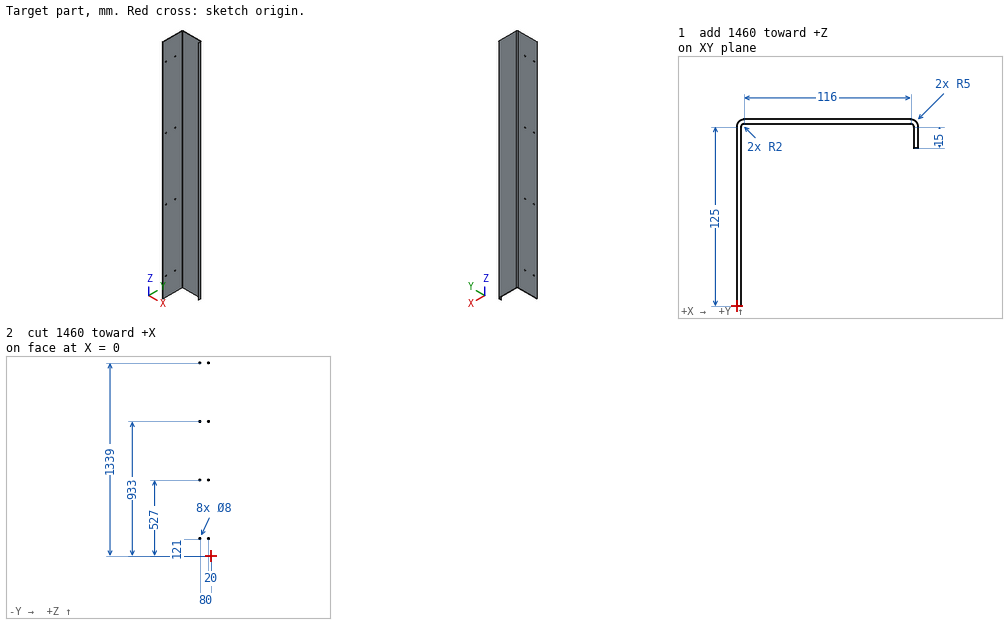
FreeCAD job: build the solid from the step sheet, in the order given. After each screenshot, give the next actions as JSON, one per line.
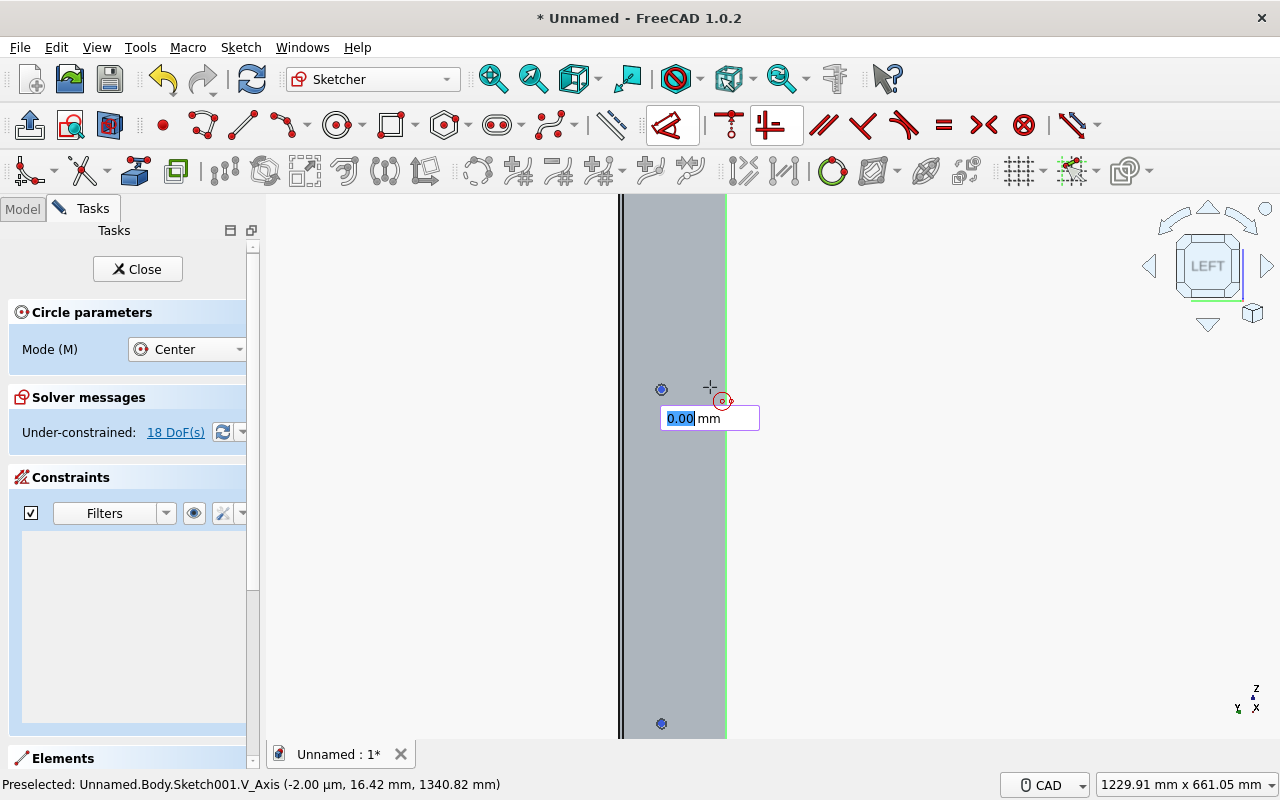
{"action": "scroll", "coordinate": [712, 384], "scroll_direction": "up", "scroll_amount": 8}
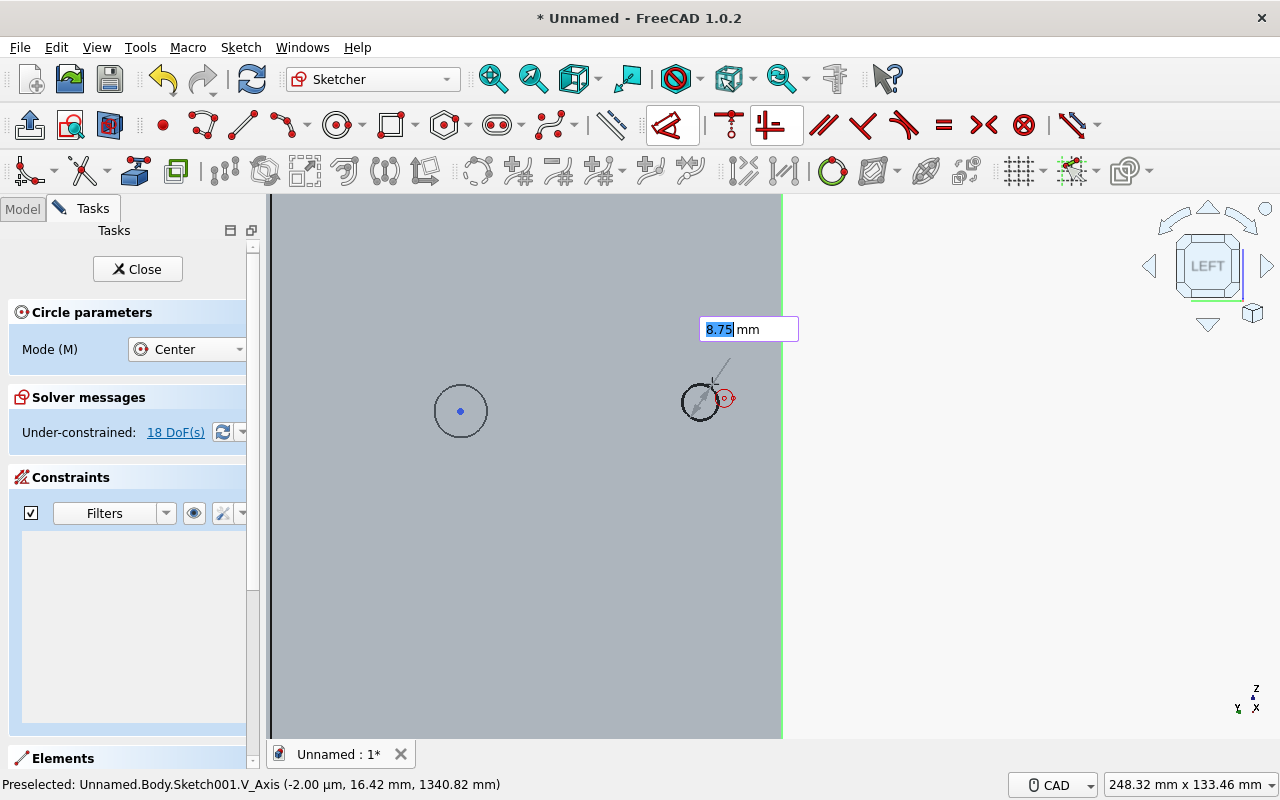
{"action": "left_click", "coordinate": [712, 385]}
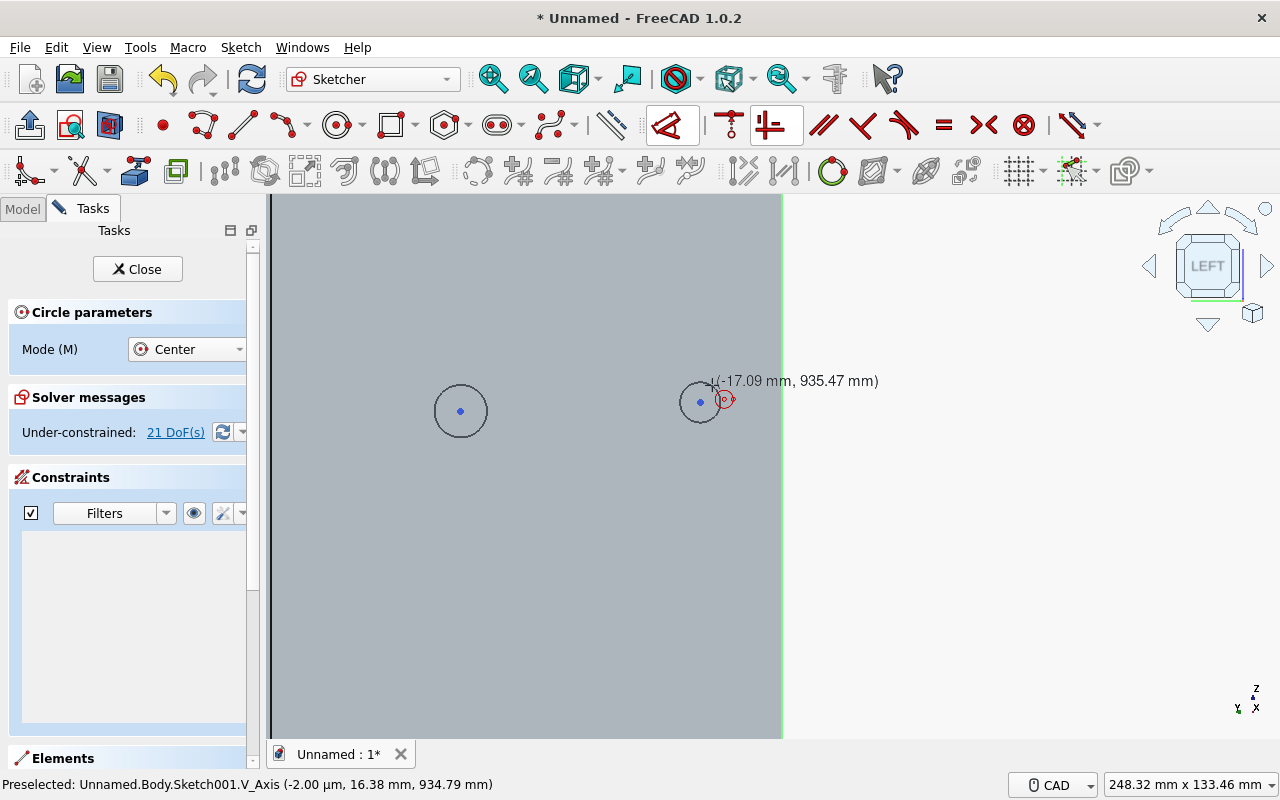
{"action": "scroll", "coordinate": [711, 402], "scroll_direction": "down", "scroll_amount": 14}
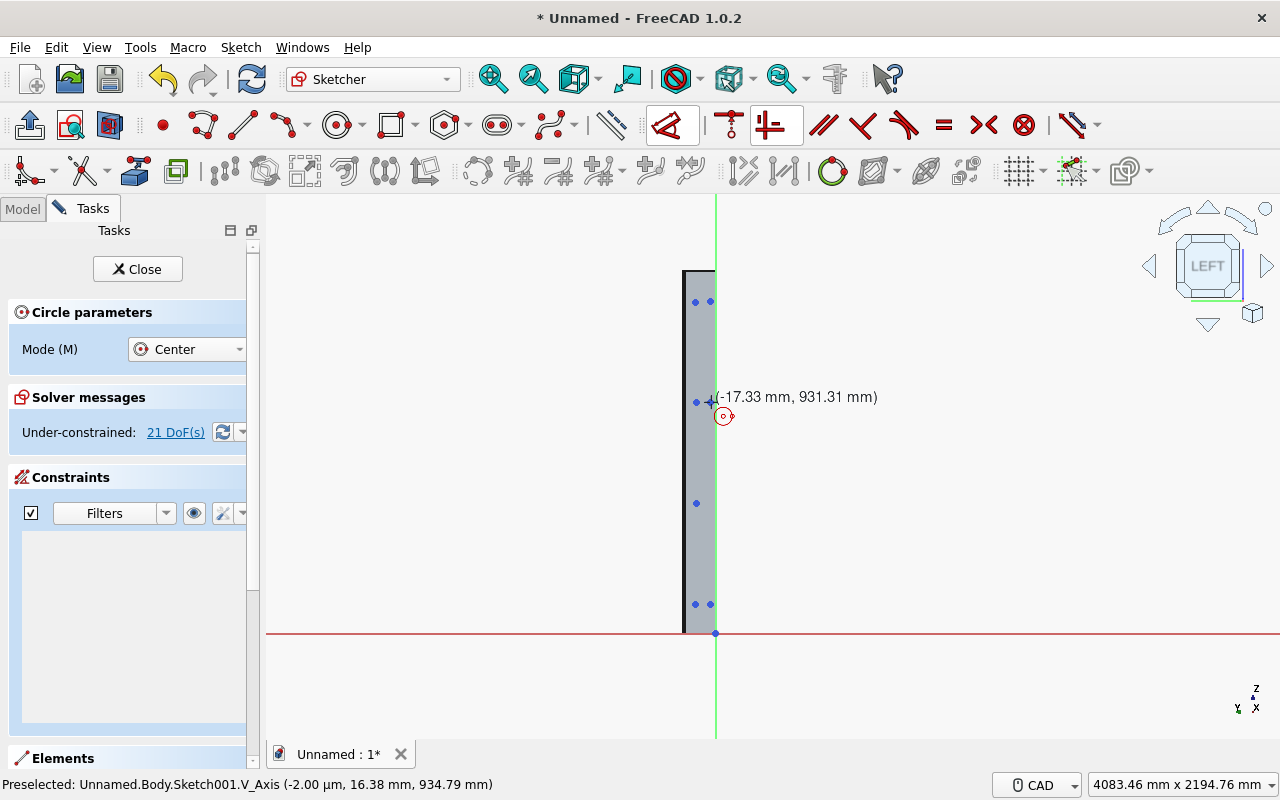
{"action": "scroll", "coordinate": [711, 503], "scroll_direction": "up", "scroll_amount": 16}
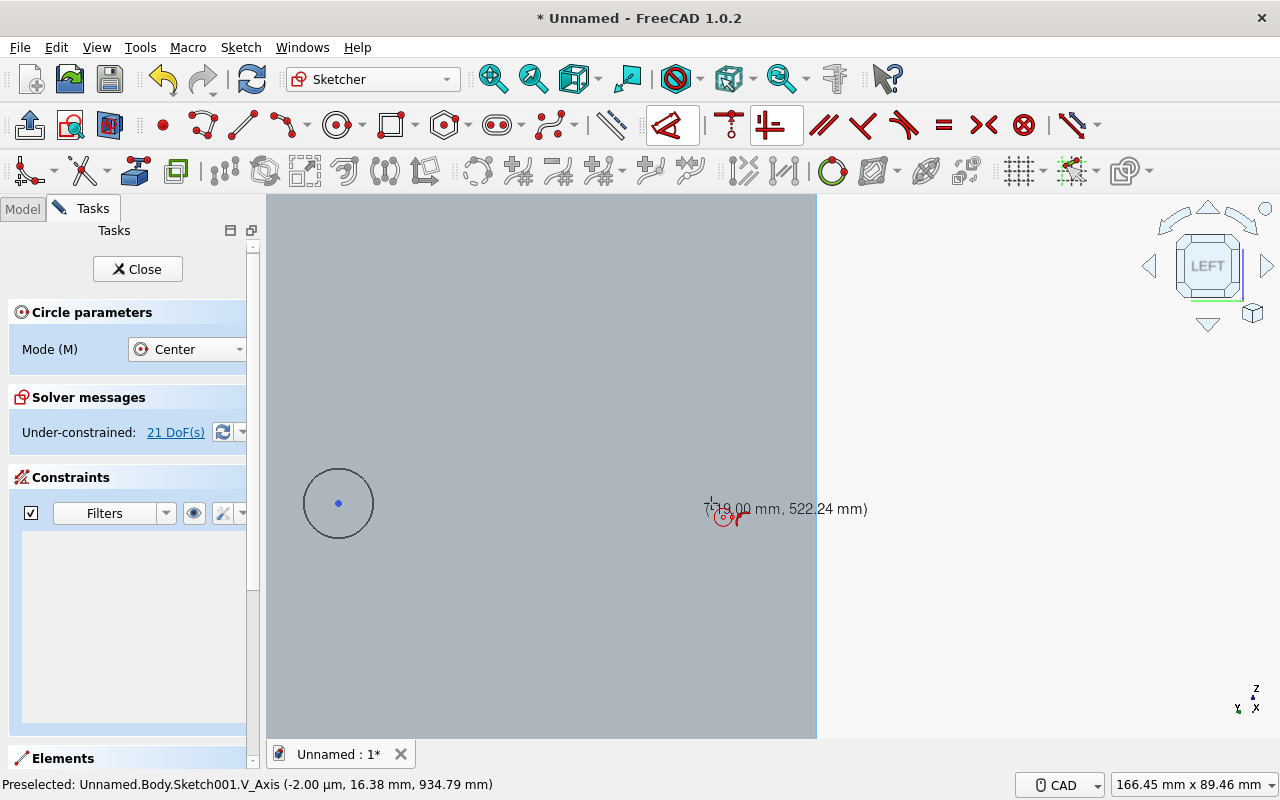
{"action": "scroll", "coordinate": [712, 512], "scroll_direction": "down", "scroll_amount": 15}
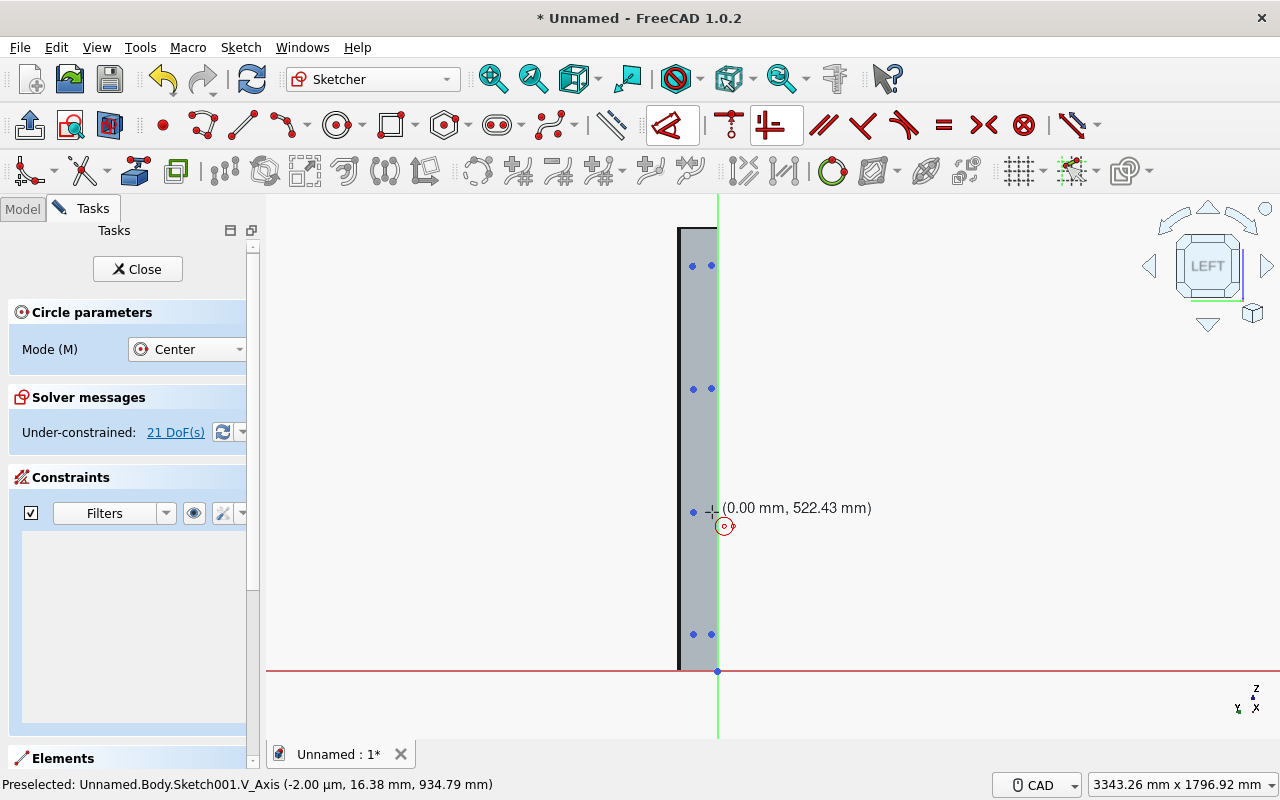
{"action": "scroll", "coordinate": [712, 511], "scroll_direction": "up", "scroll_amount": 5}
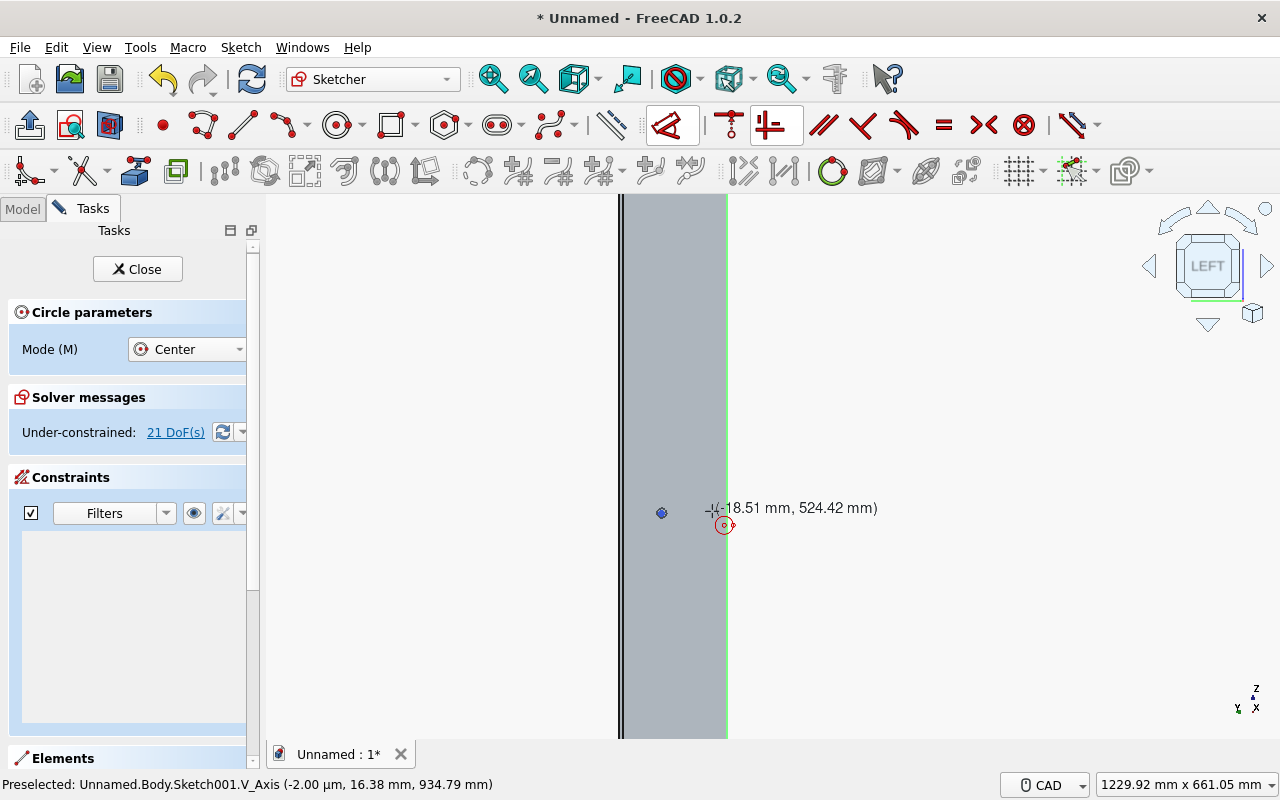
{"action": "left_click", "coordinate": [710, 511]}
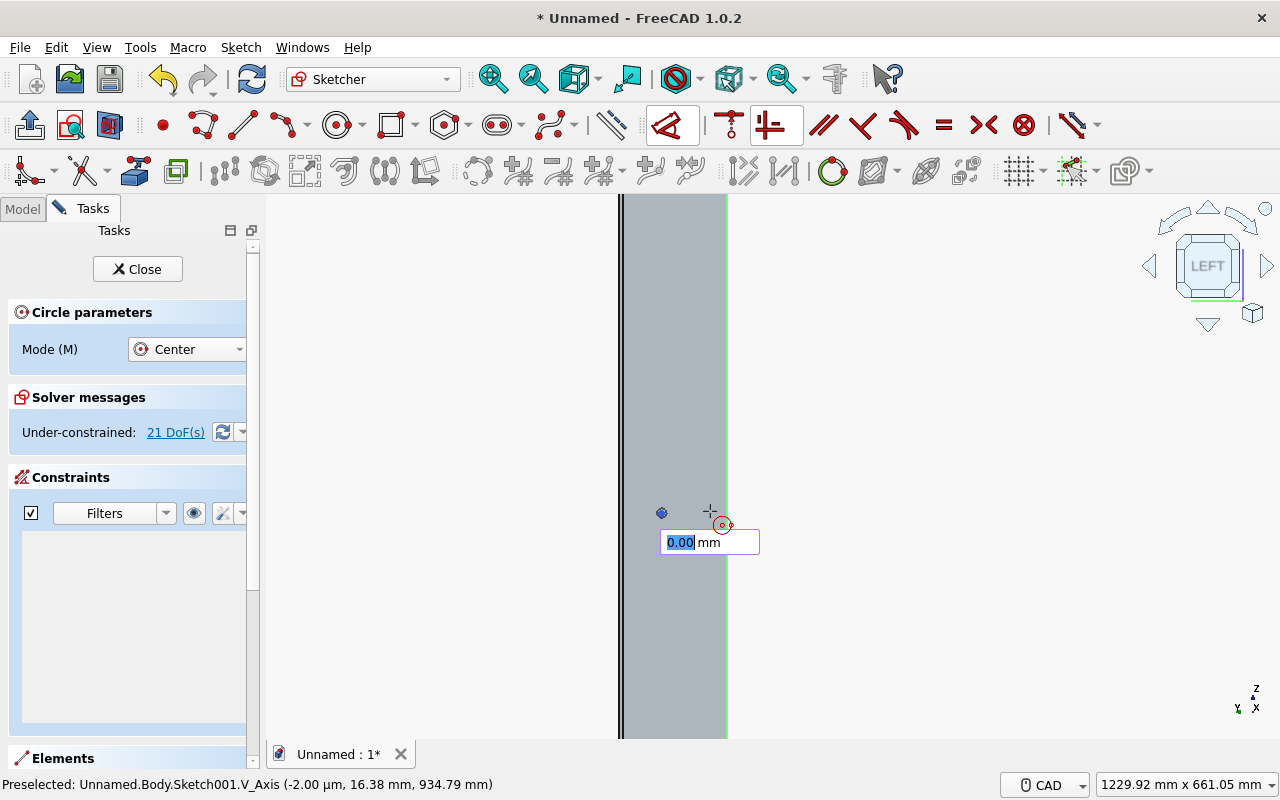
{"action": "scroll", "coordinate": [712, 508], "scroll_direction": "up", "scroll_amount": 8}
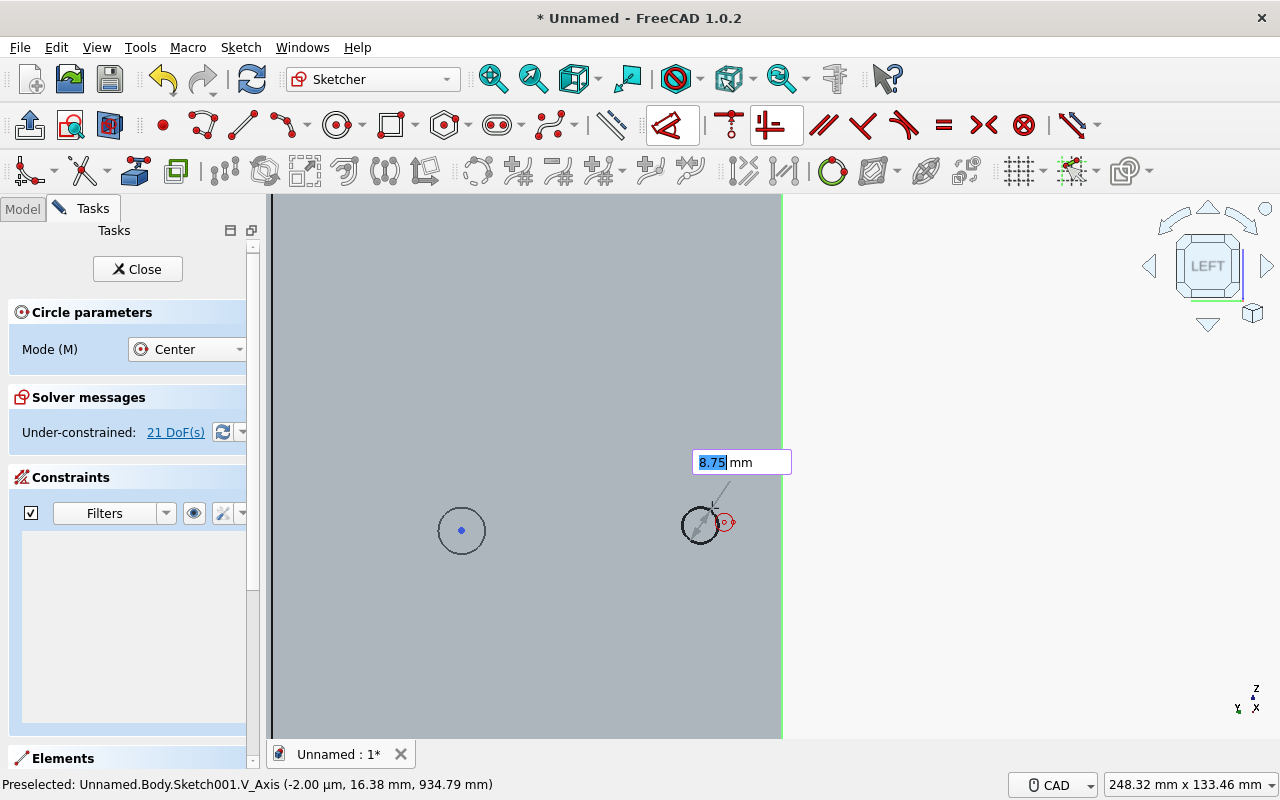
{"action": "left_click", "coordinate": [712, 507]}
{"action": "key", "text": "Escape"}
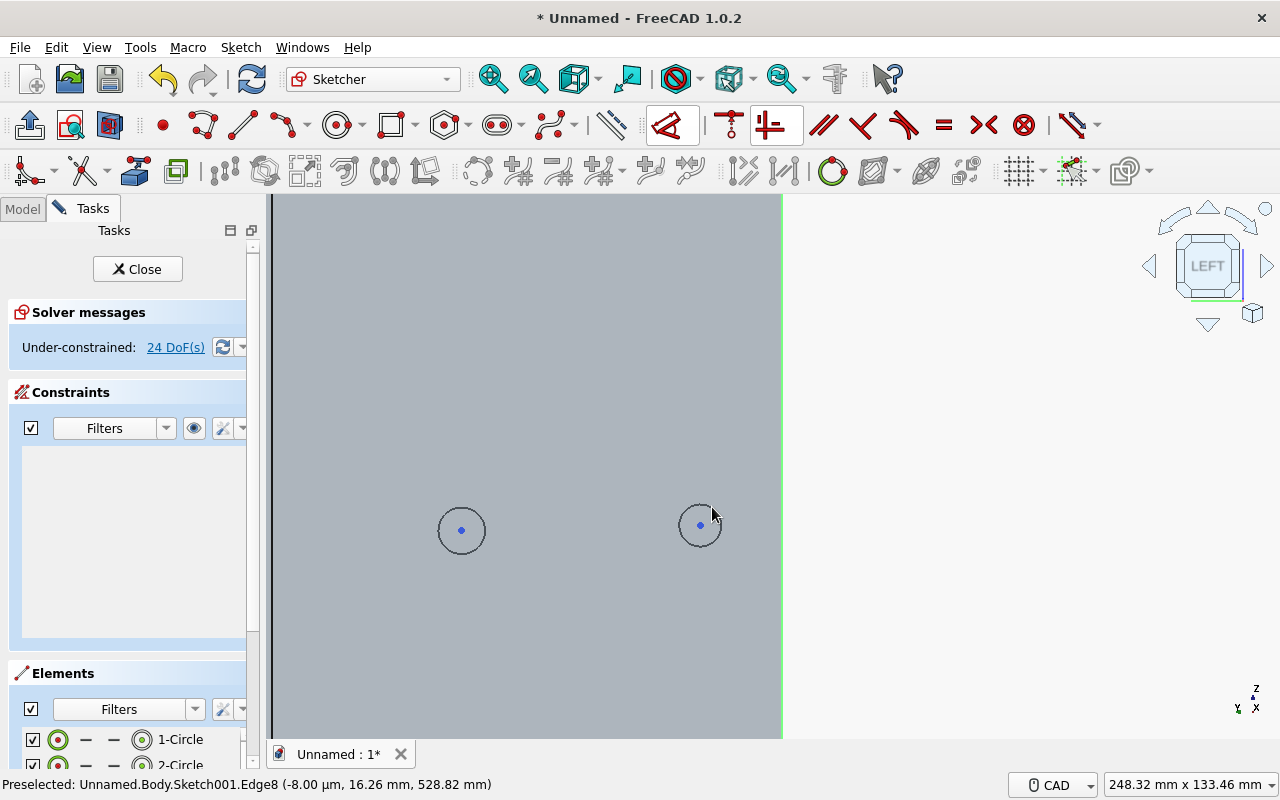
{"action": "scroll", "coordinate": [711, 501], "scroll_direction": "down", "scroll_amount": 14}